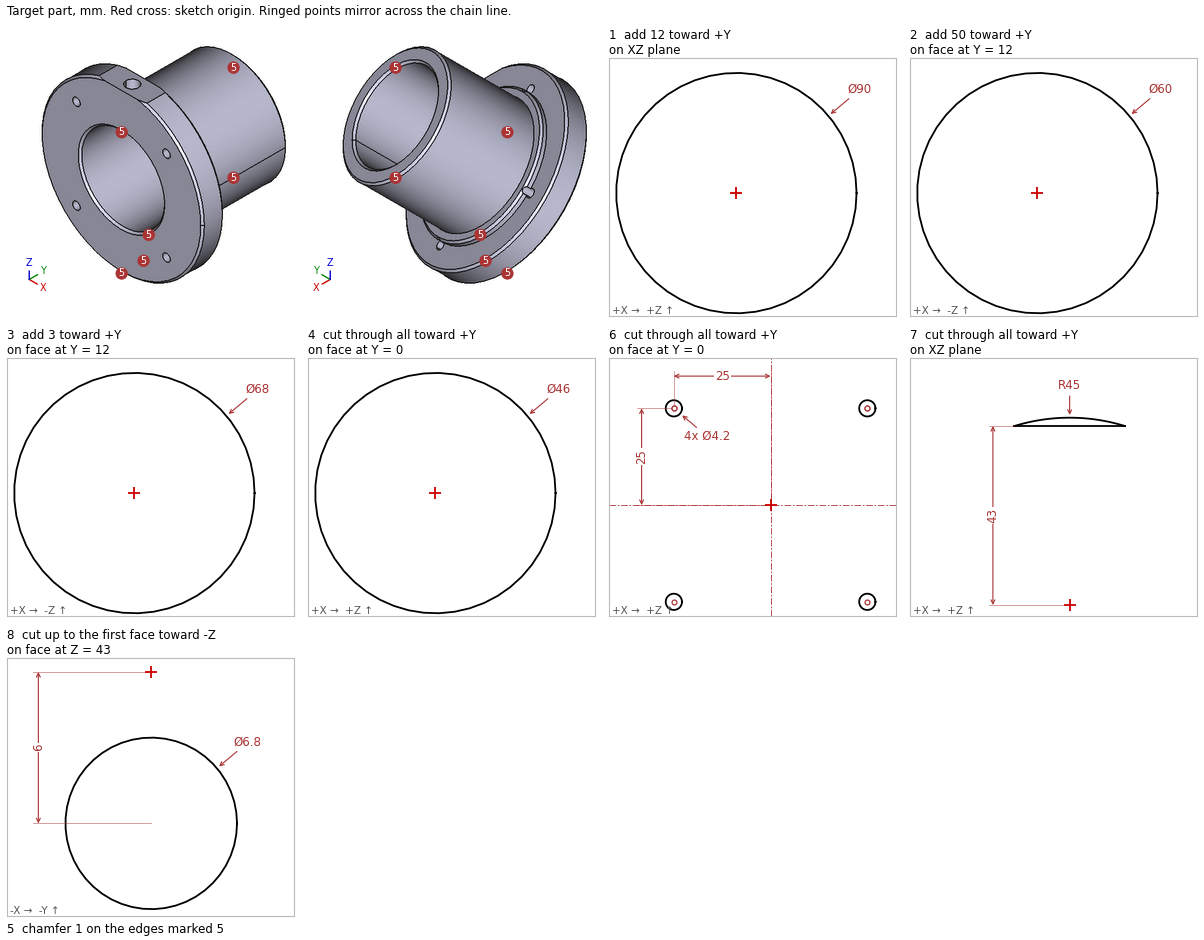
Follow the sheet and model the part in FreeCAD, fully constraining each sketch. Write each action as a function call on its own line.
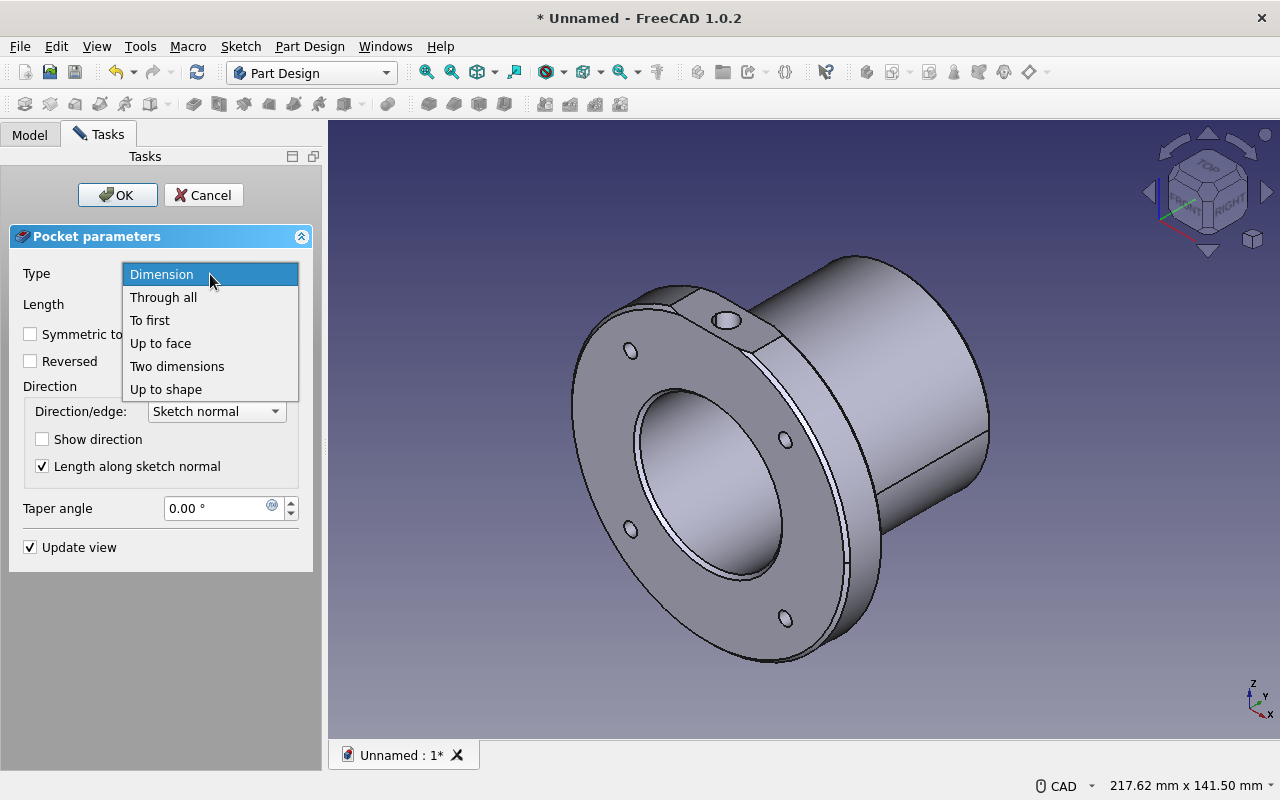
click(208, 320)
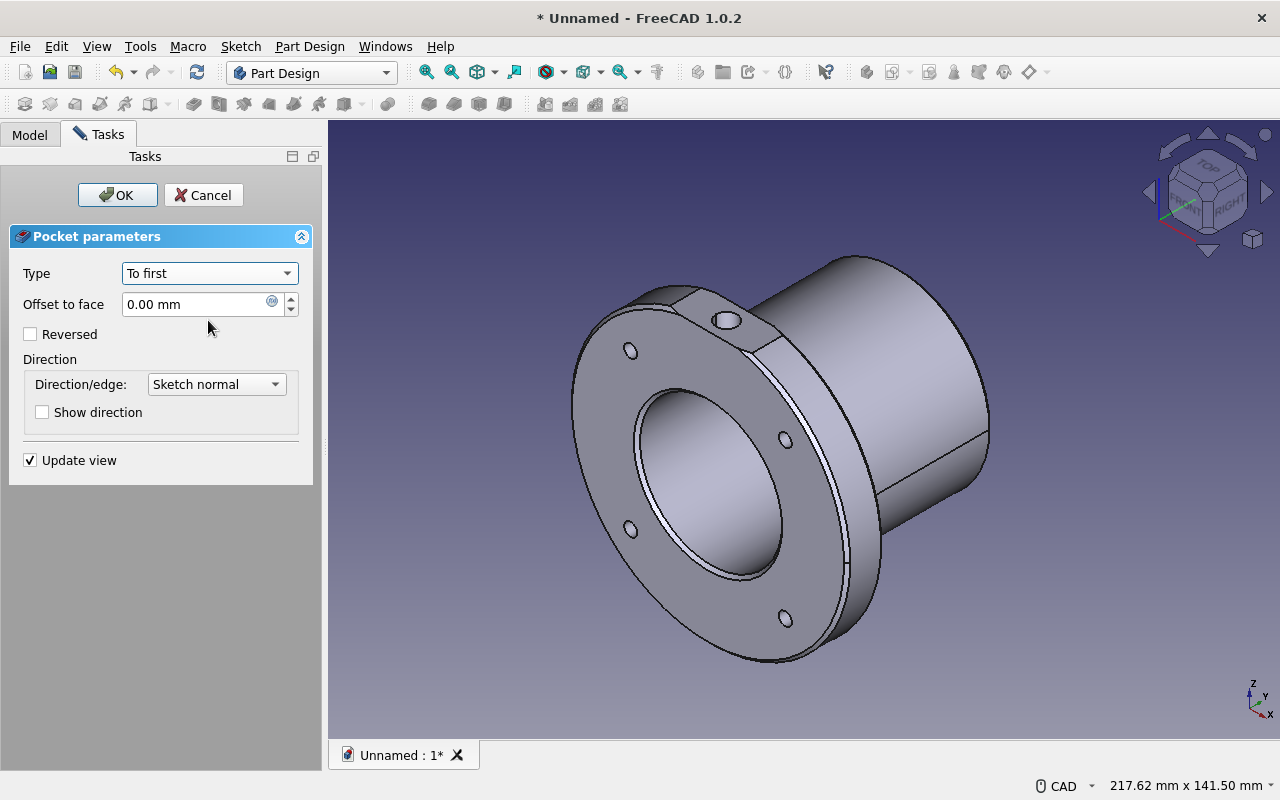
click(118, 195)